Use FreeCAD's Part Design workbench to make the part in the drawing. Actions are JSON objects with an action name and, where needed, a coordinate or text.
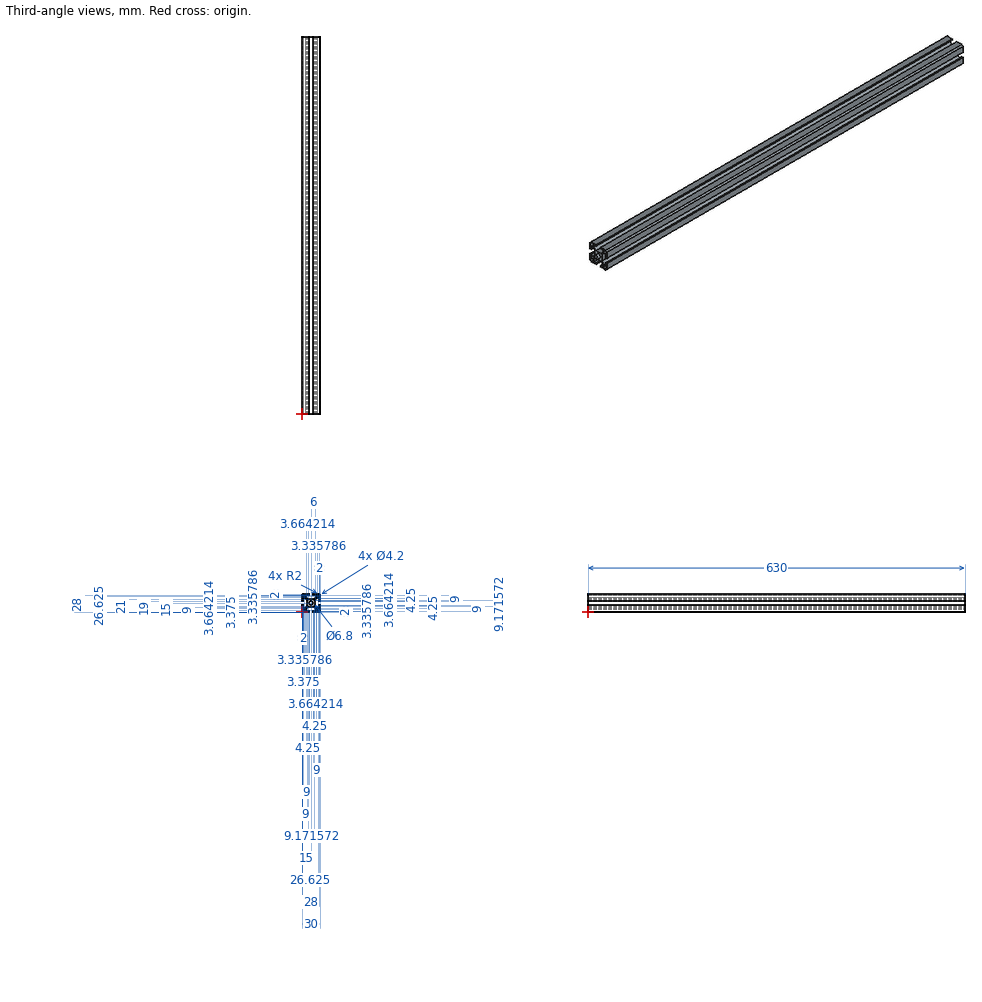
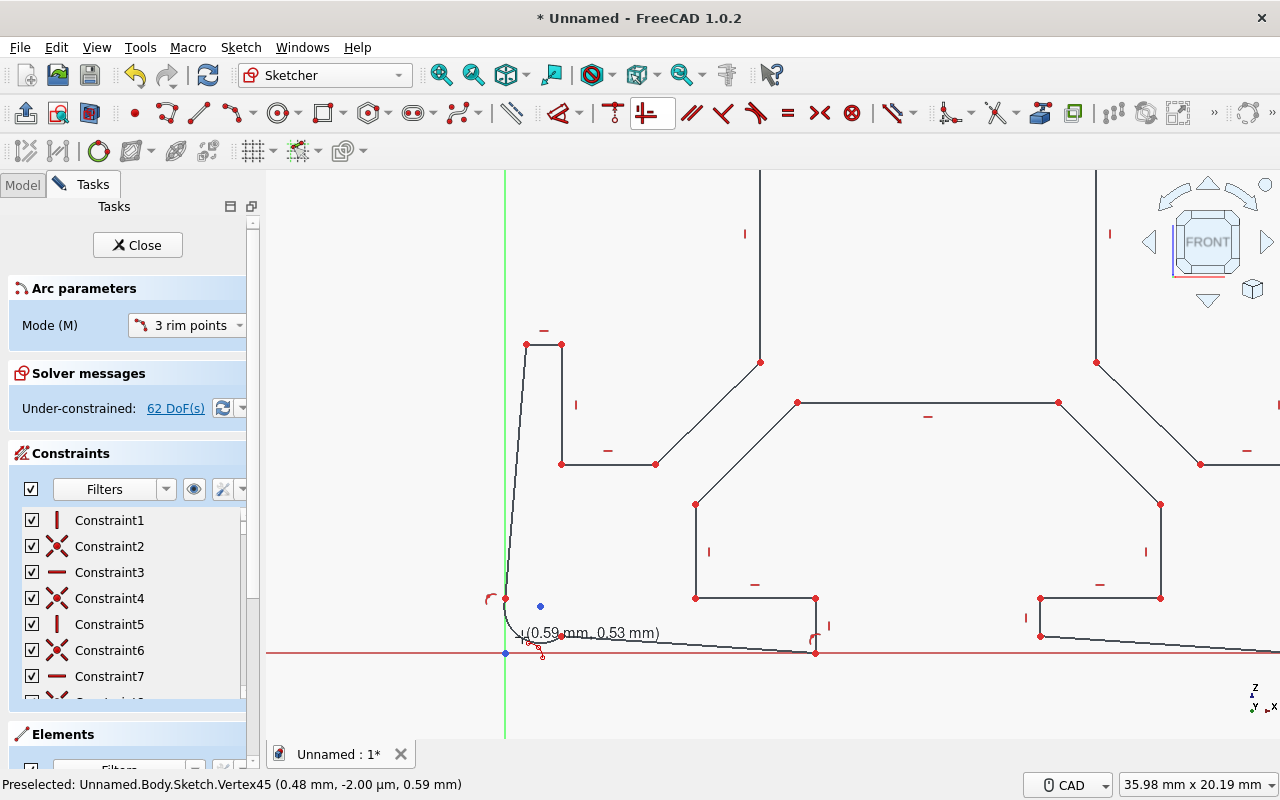
{"action": "scroll", "coordinate": [522, 637], "scroll_direction": "down", "scroll_amount": 4}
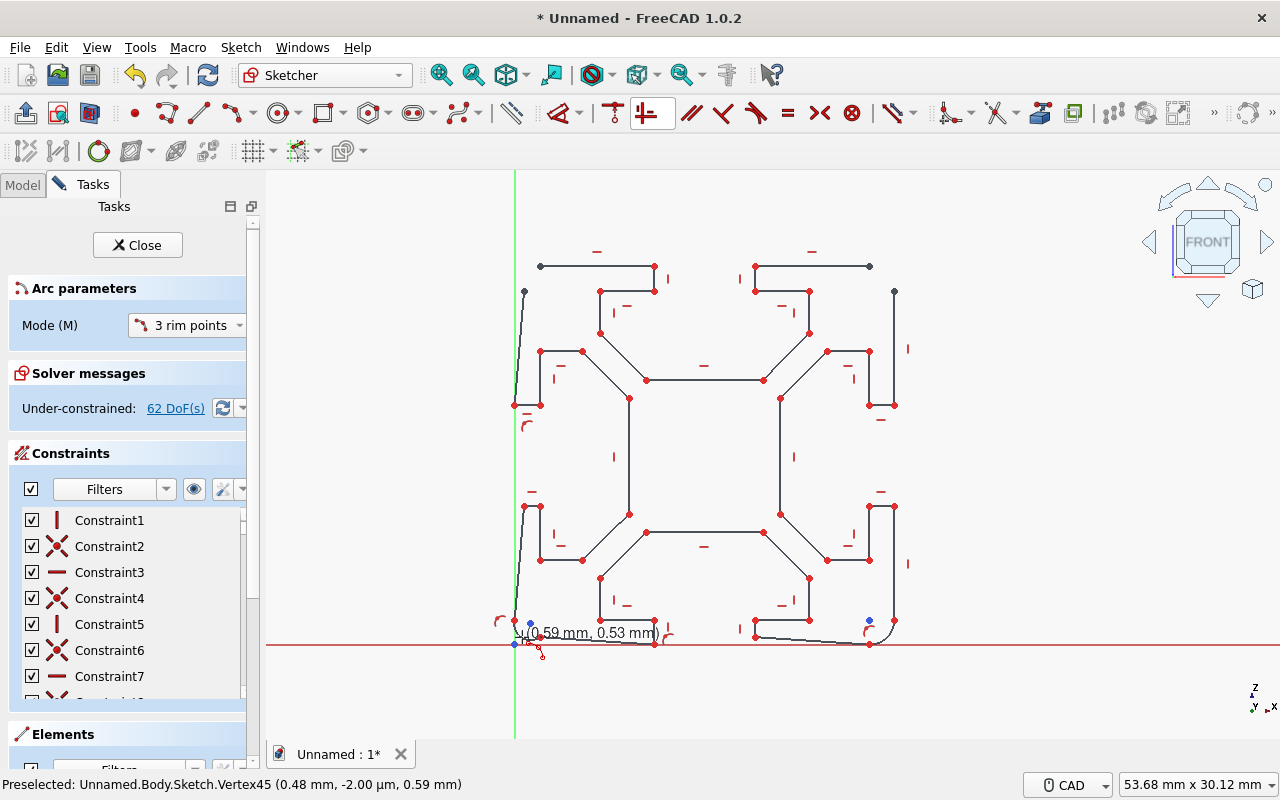
{"action": "left_click", "coordinate": [524, 291]}
{"action": "left_click", "coordinate": [540, 266]}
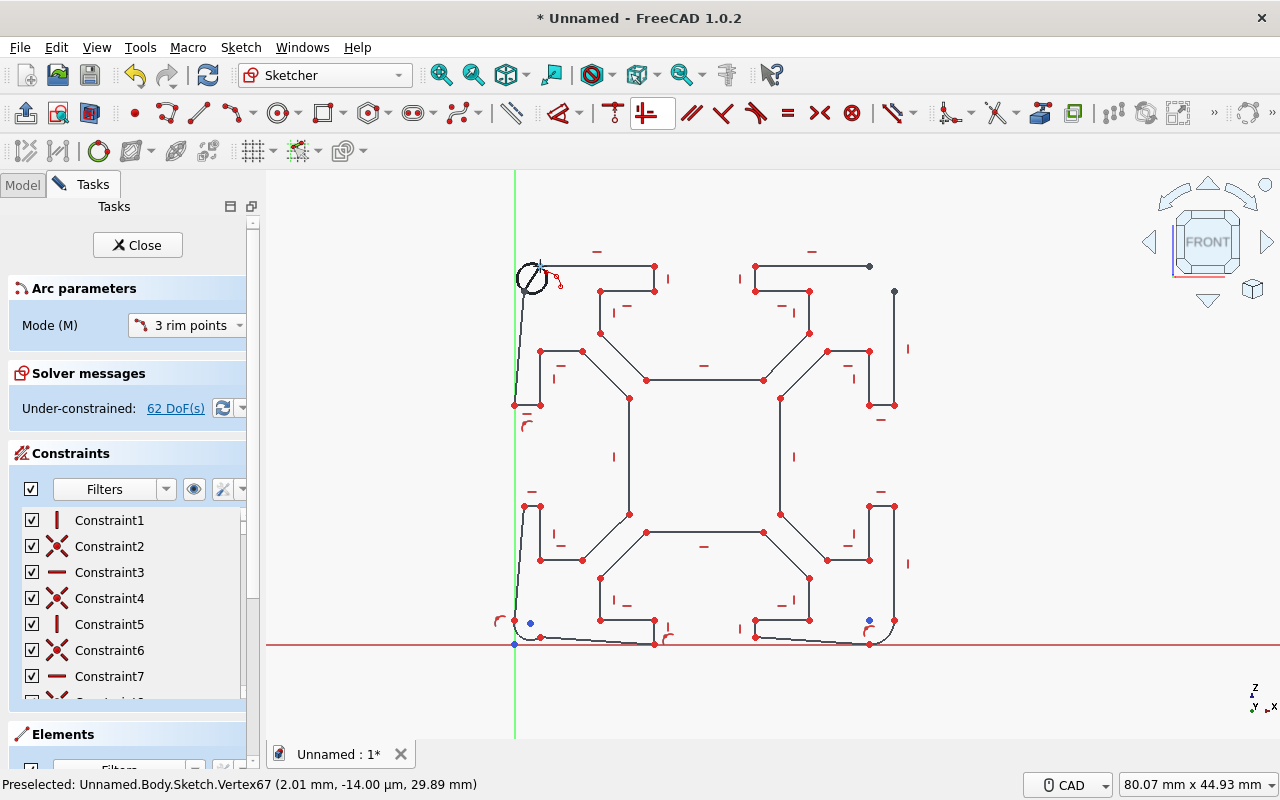
{"action": "scroll", "coordinate": [522, 272], "scroll_direction": "up", "scroll_amount": 4}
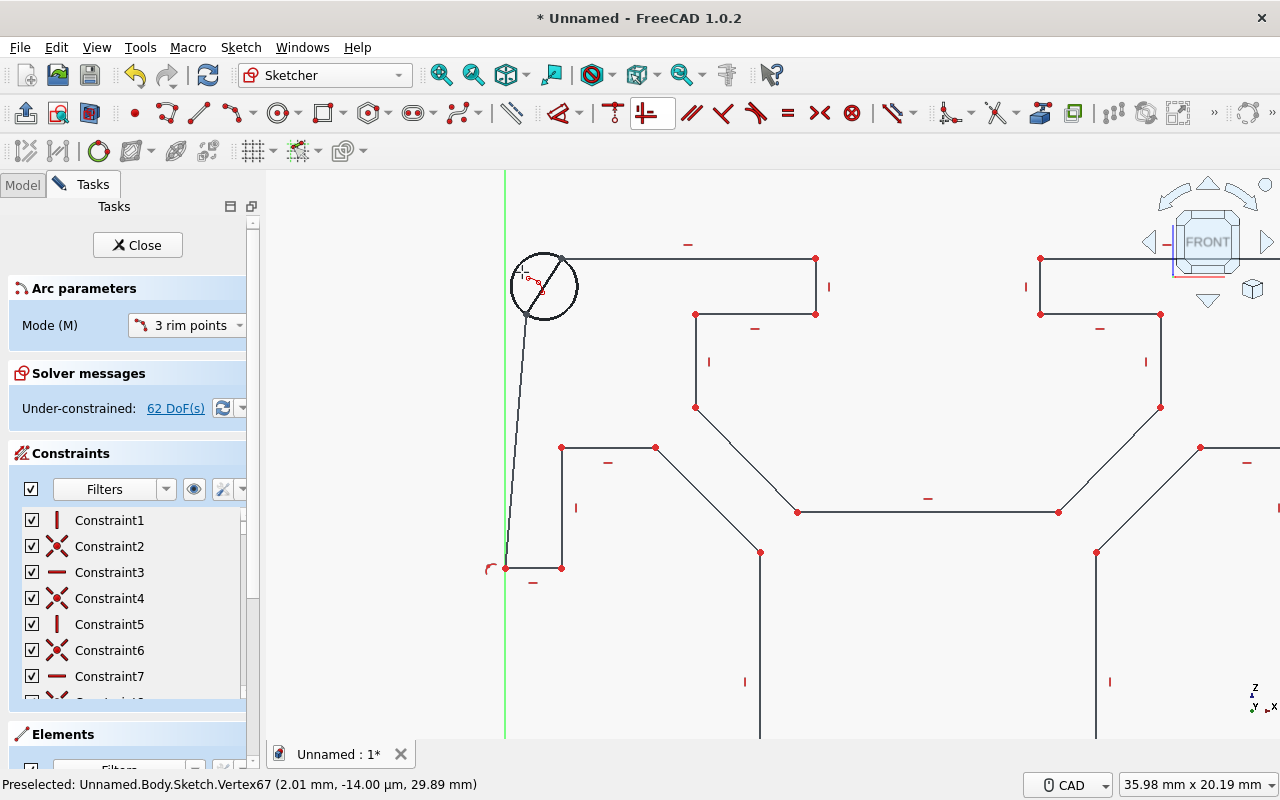
{"action": "left_click", "coordinate": [522, 272]}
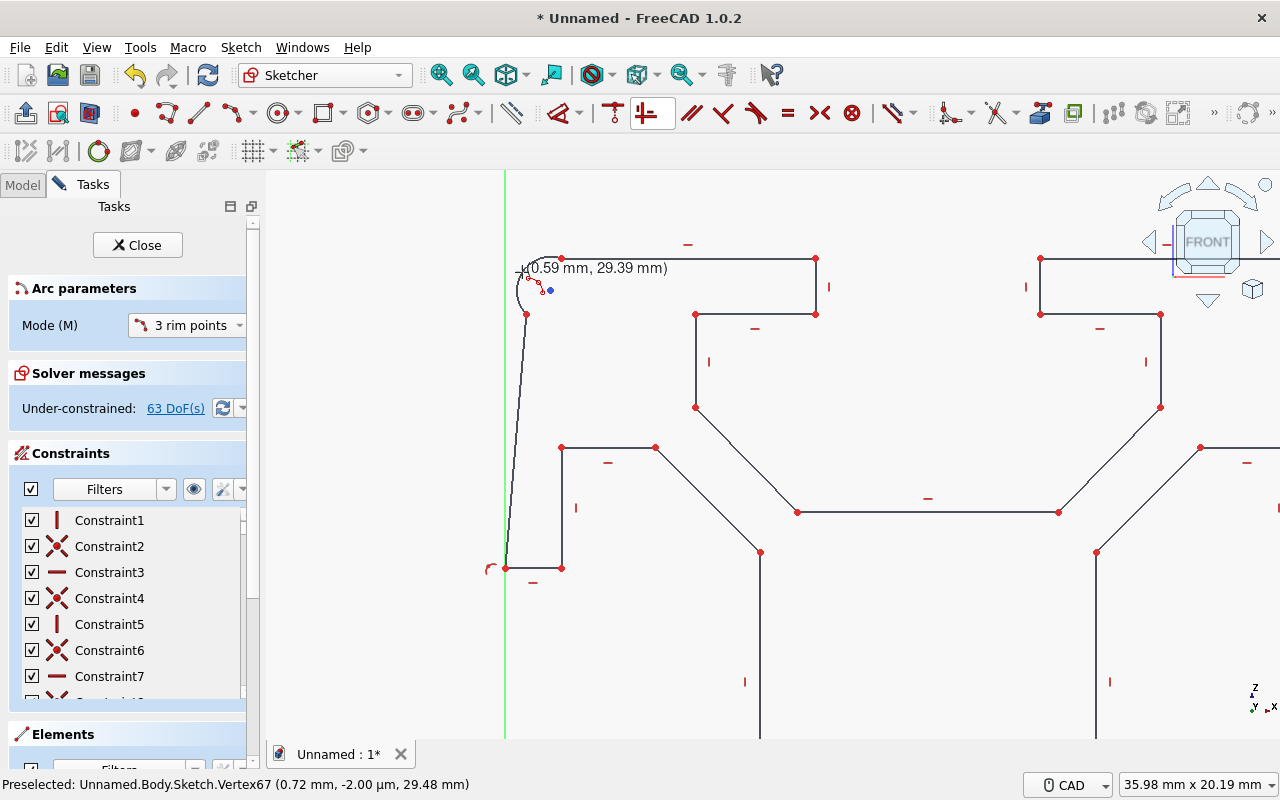
{"action": "scroll", "coordinate": [522, 272], "scroll_direction": "down", "scroll_amount": 4}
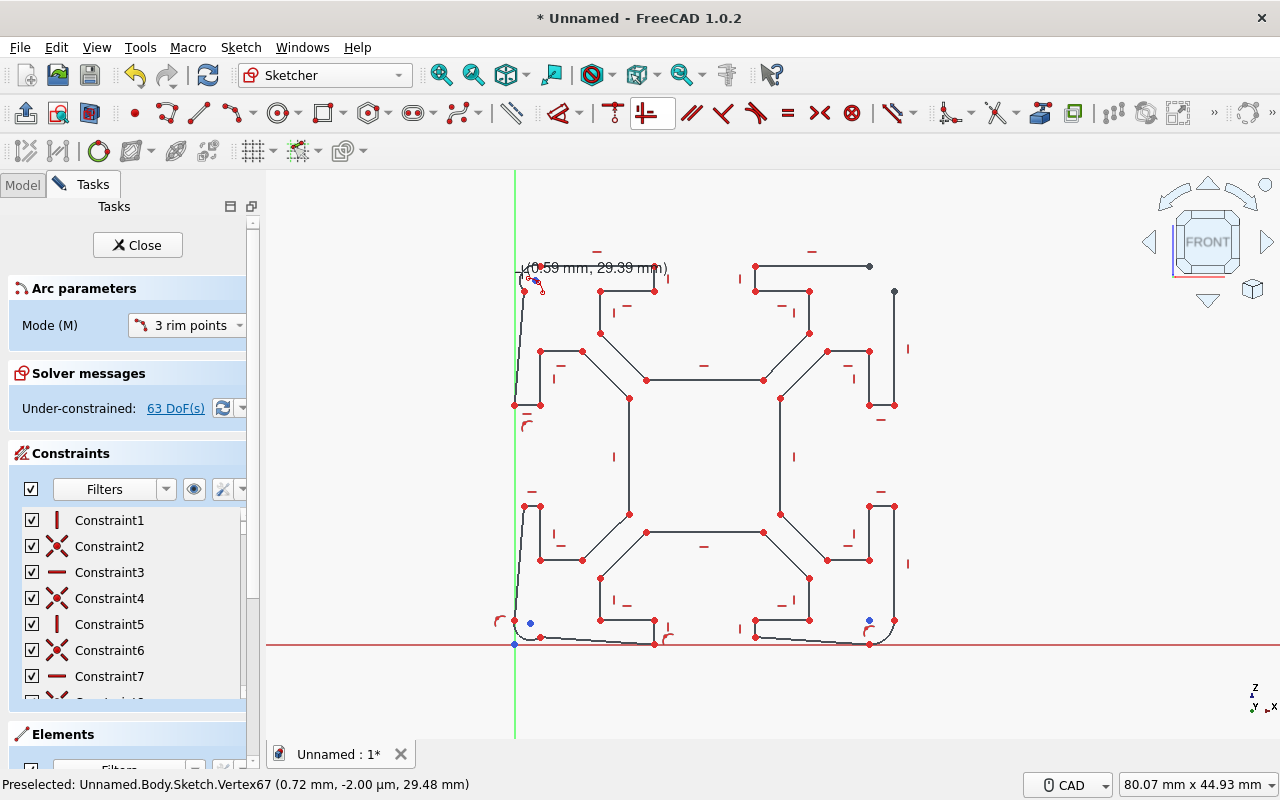
{"action": "left_click", "coordinate": [869, 266]}
{"action": "left_click", "coordinate": [894, 291]}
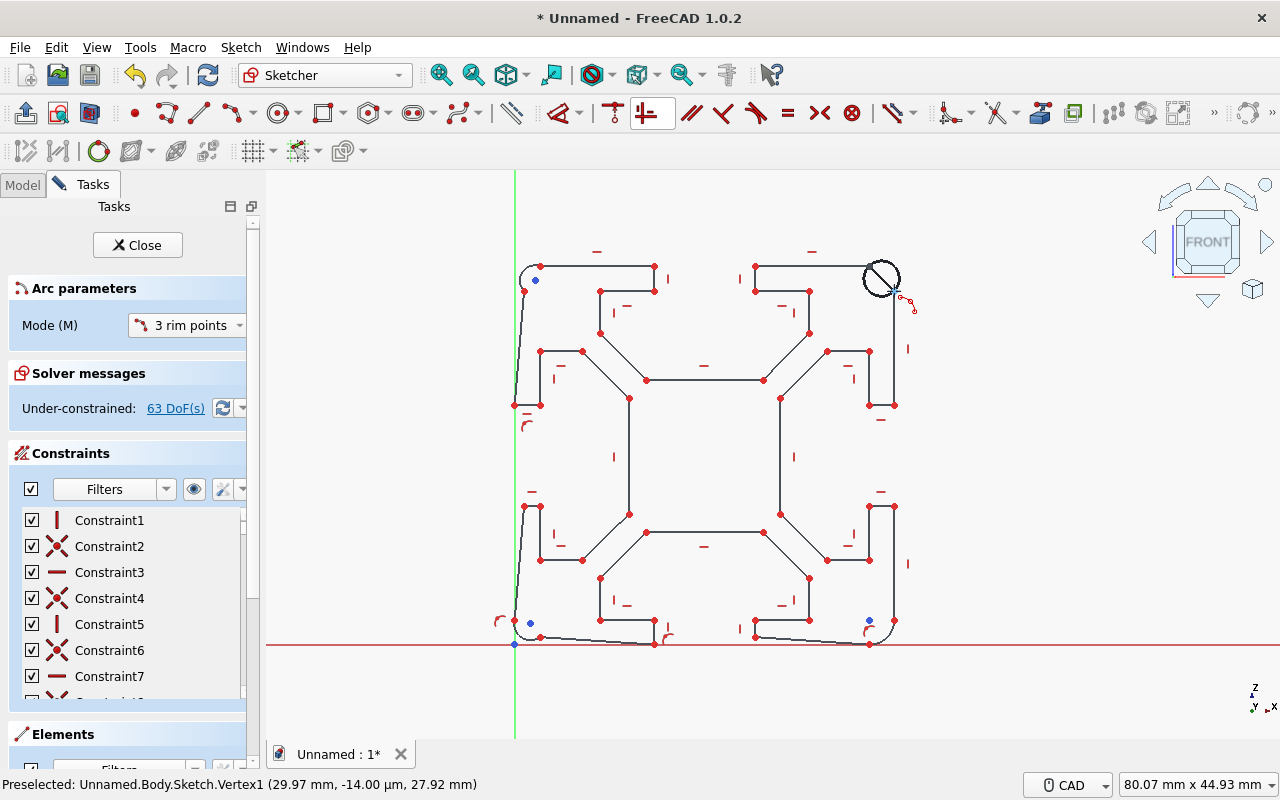
{"action": "scroll", "coordinate": [887, 272], "scroll_direction": "up", "scroll_amount": 4}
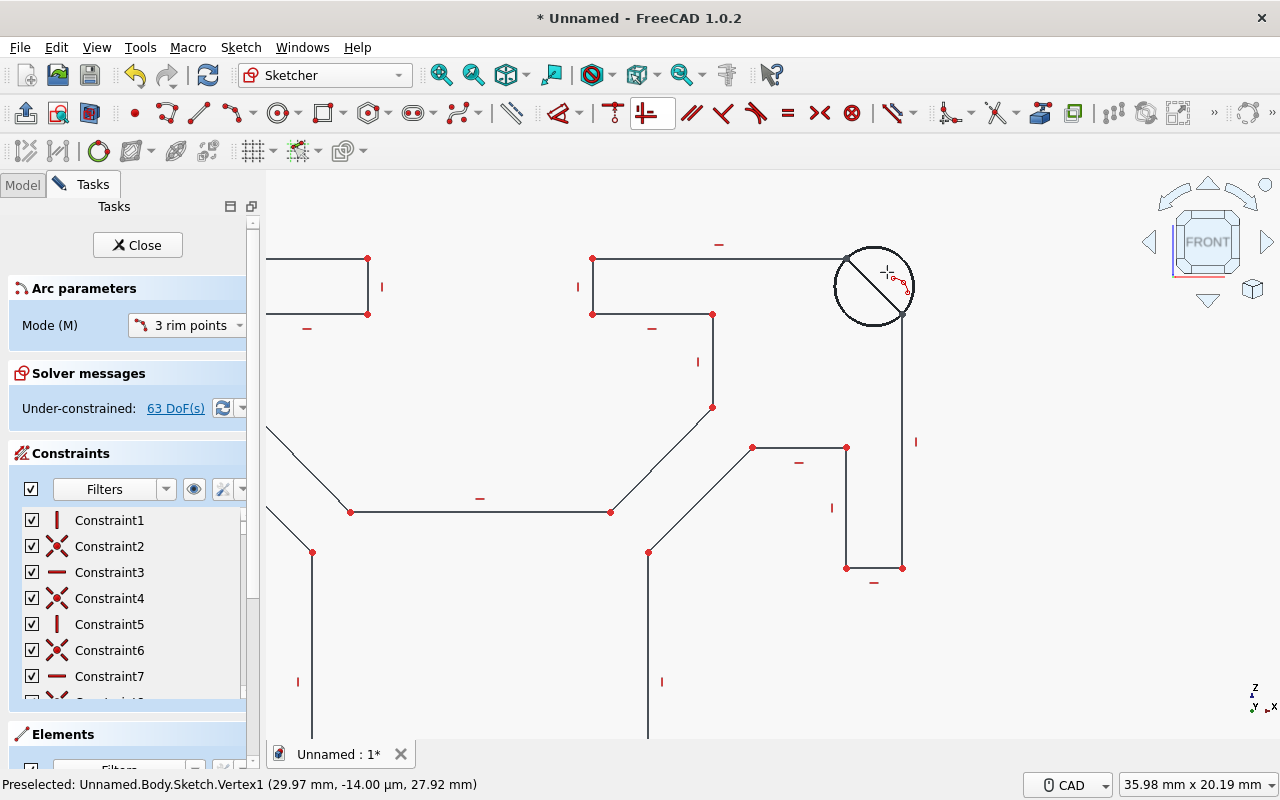
{"action": "left_click", "coordinate": [887, 272]}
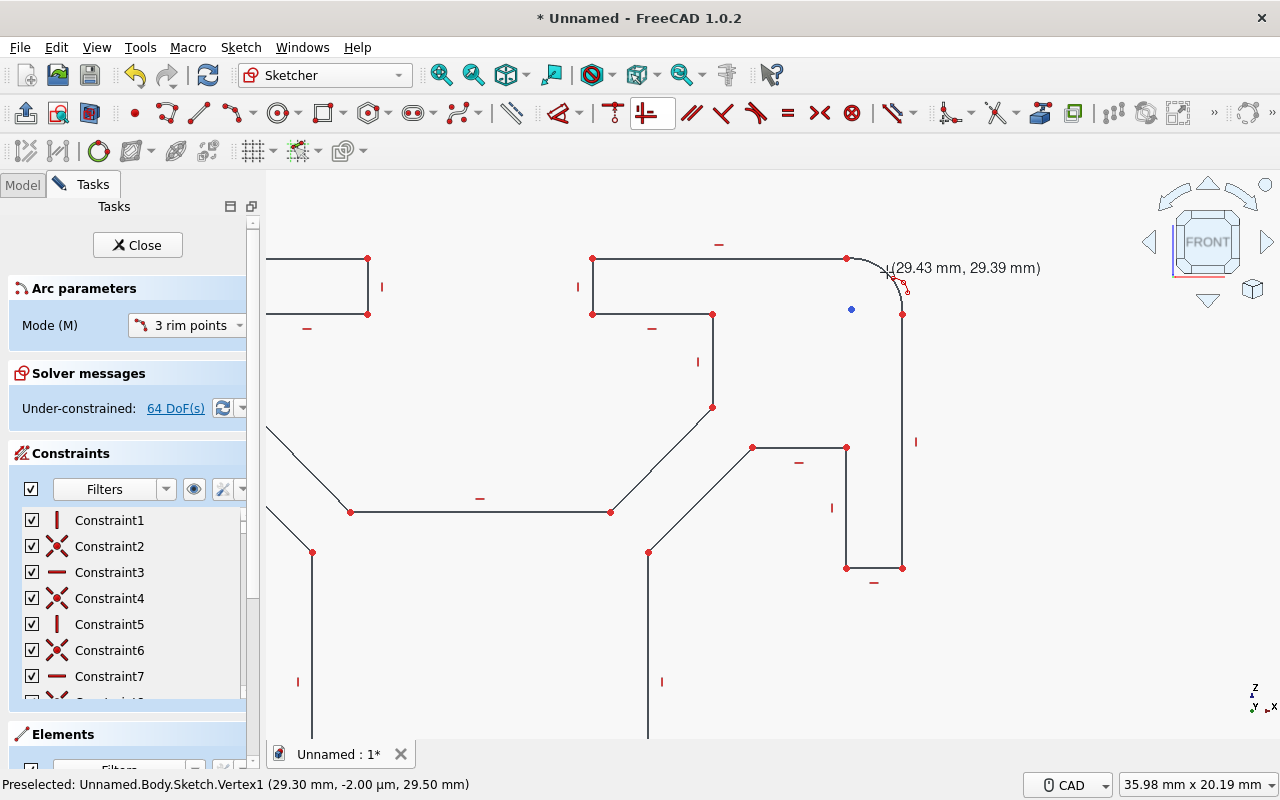
{"action": "left_click", "coordinate": [278, 114]}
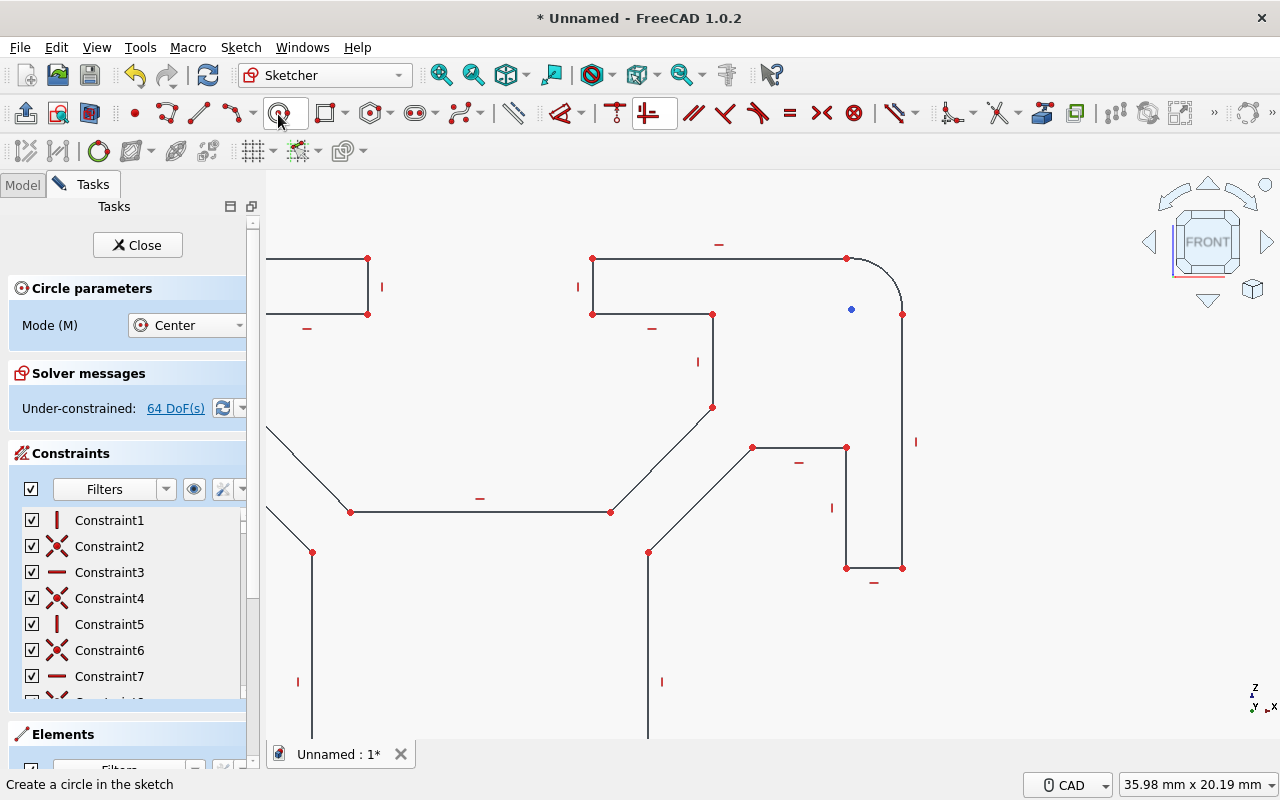
{"action": "left_click", "coordinate": [808, 351]}
{"action": "mouse_move", "coordinate": [766, 309]}